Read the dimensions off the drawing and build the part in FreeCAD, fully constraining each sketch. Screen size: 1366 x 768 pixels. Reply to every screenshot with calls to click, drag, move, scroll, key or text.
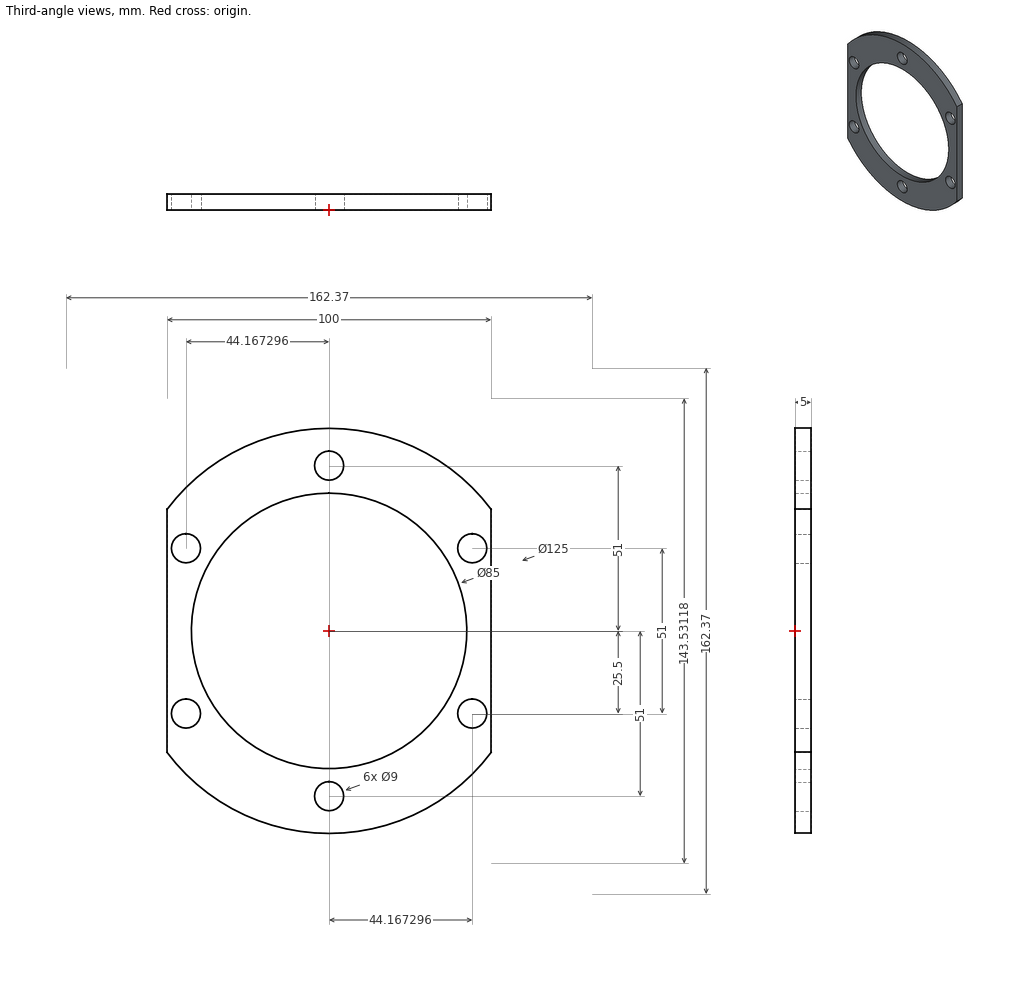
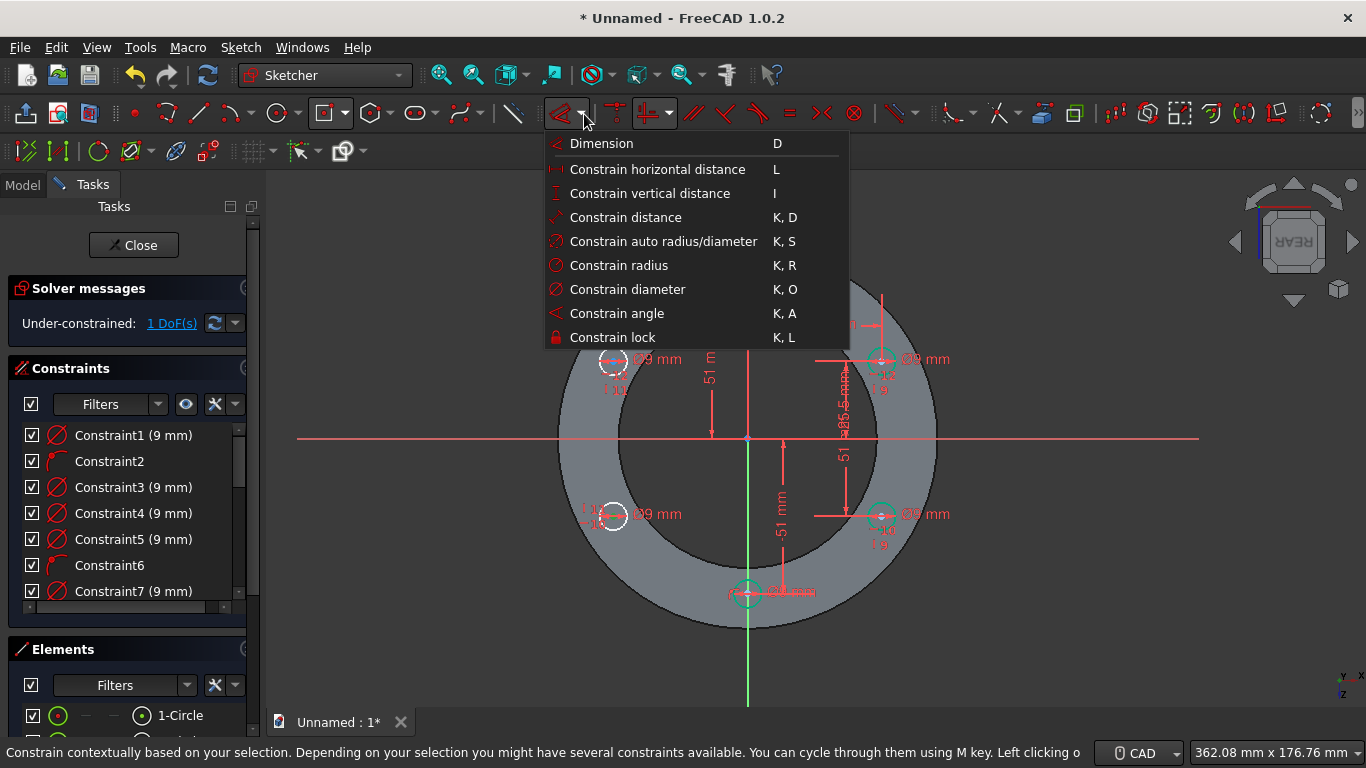
click(697, 169)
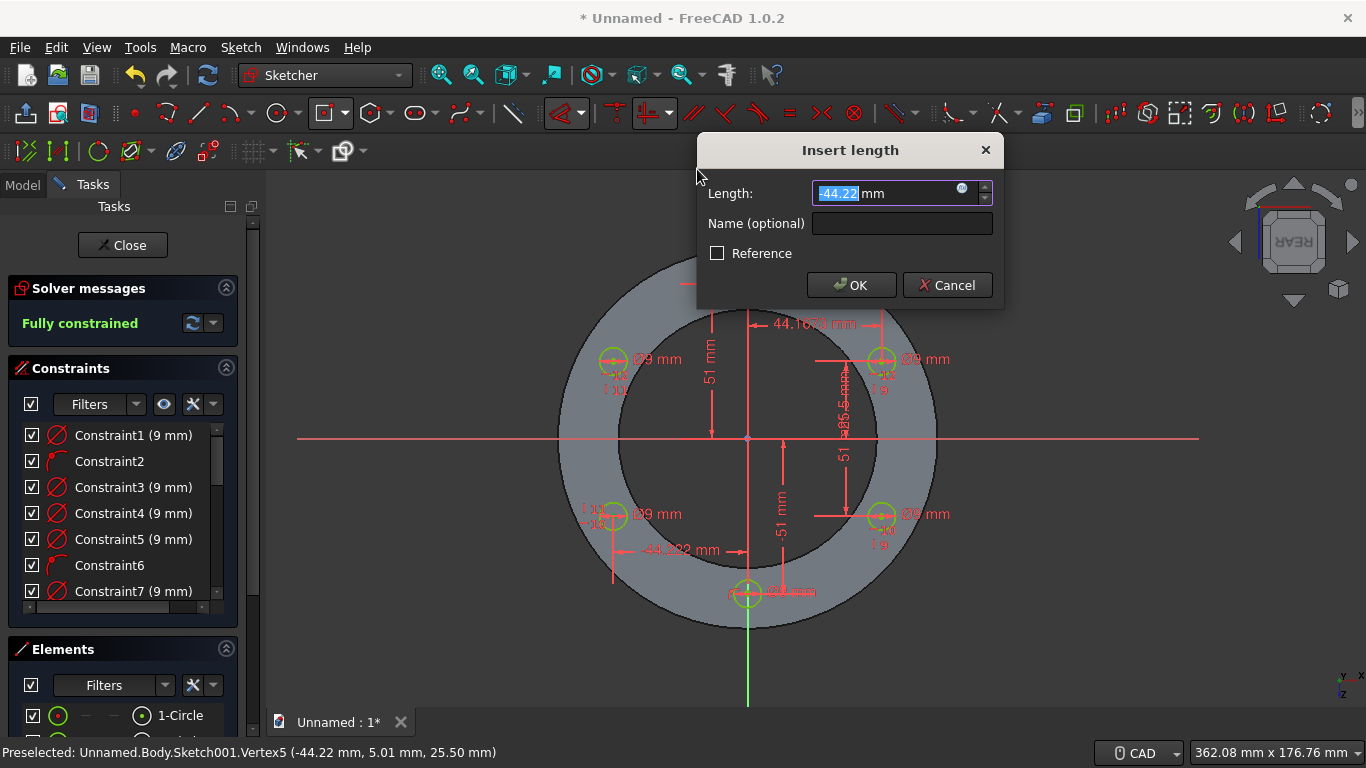
text(-44.167296)
key(Return)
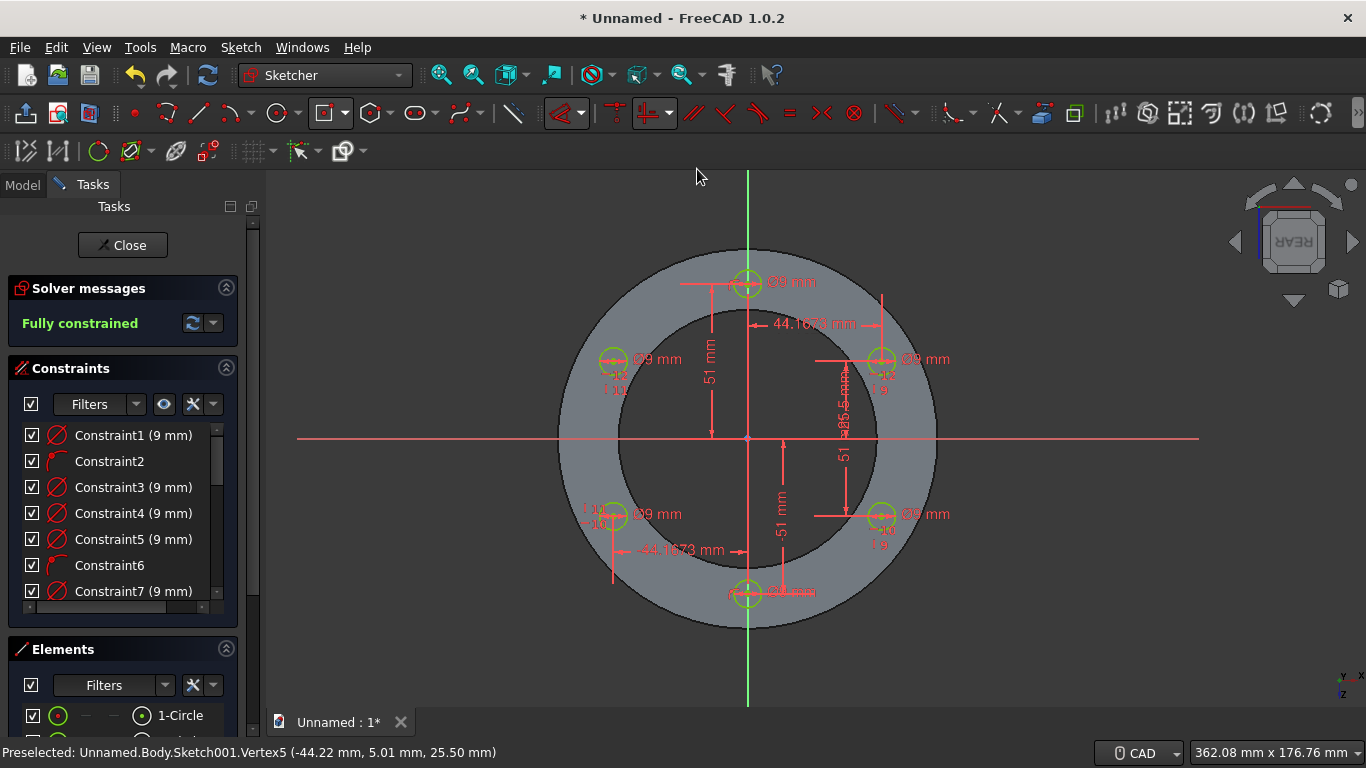
click(123, 245)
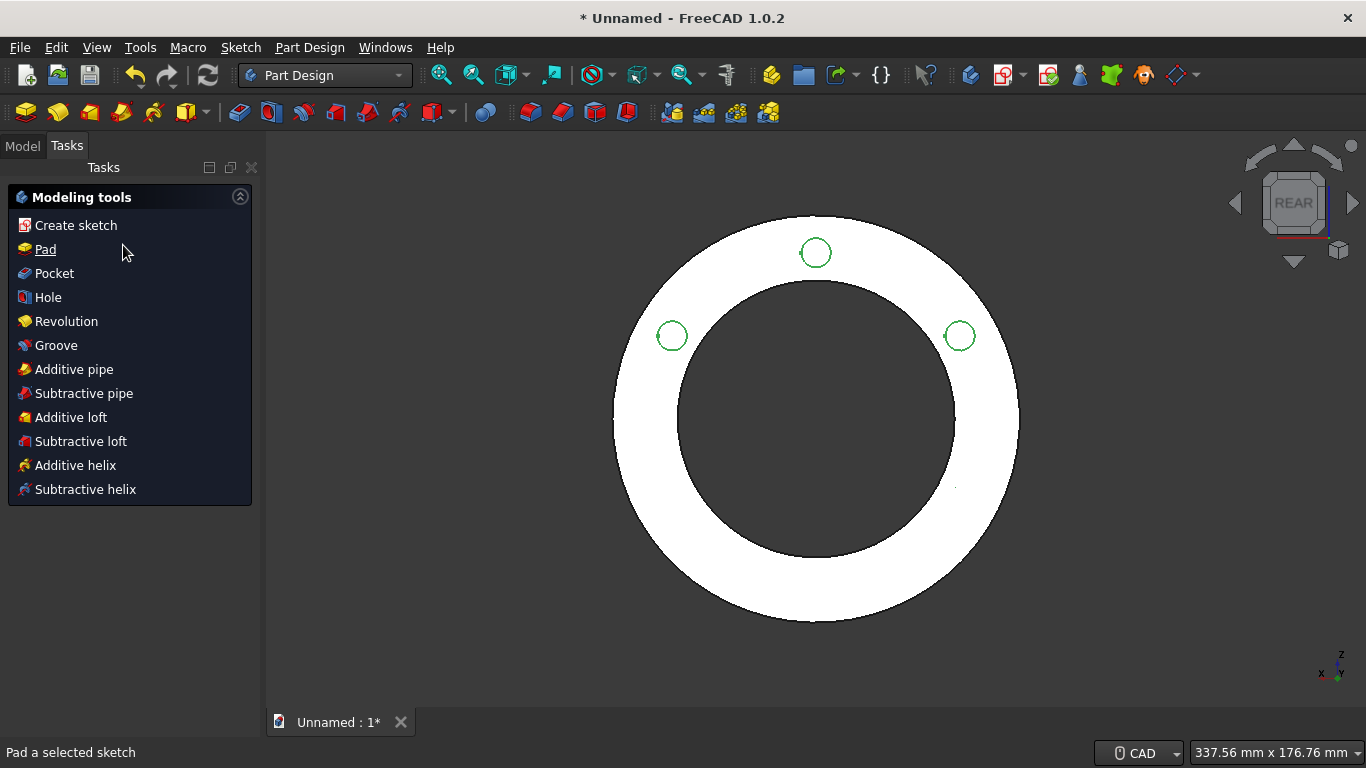
click(240, 112)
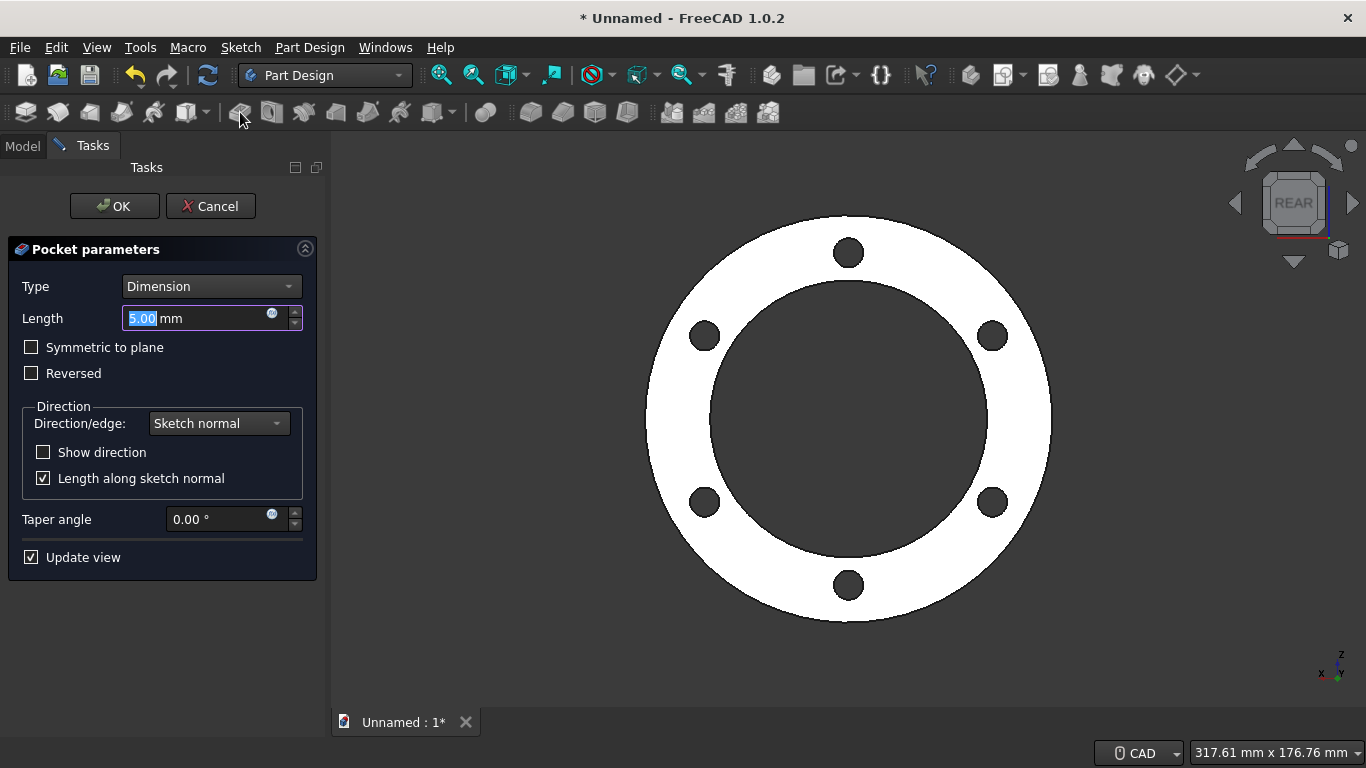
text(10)
key(Tab)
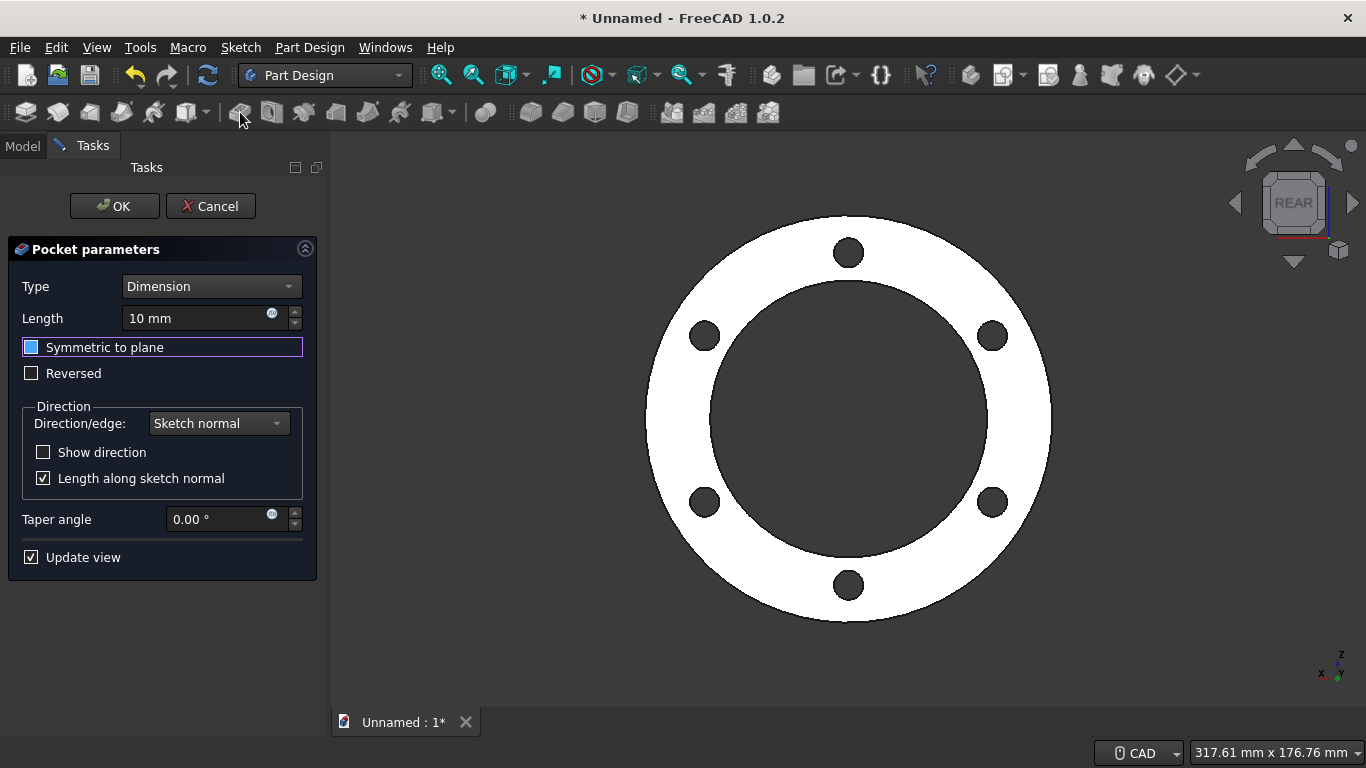
click(115, 206)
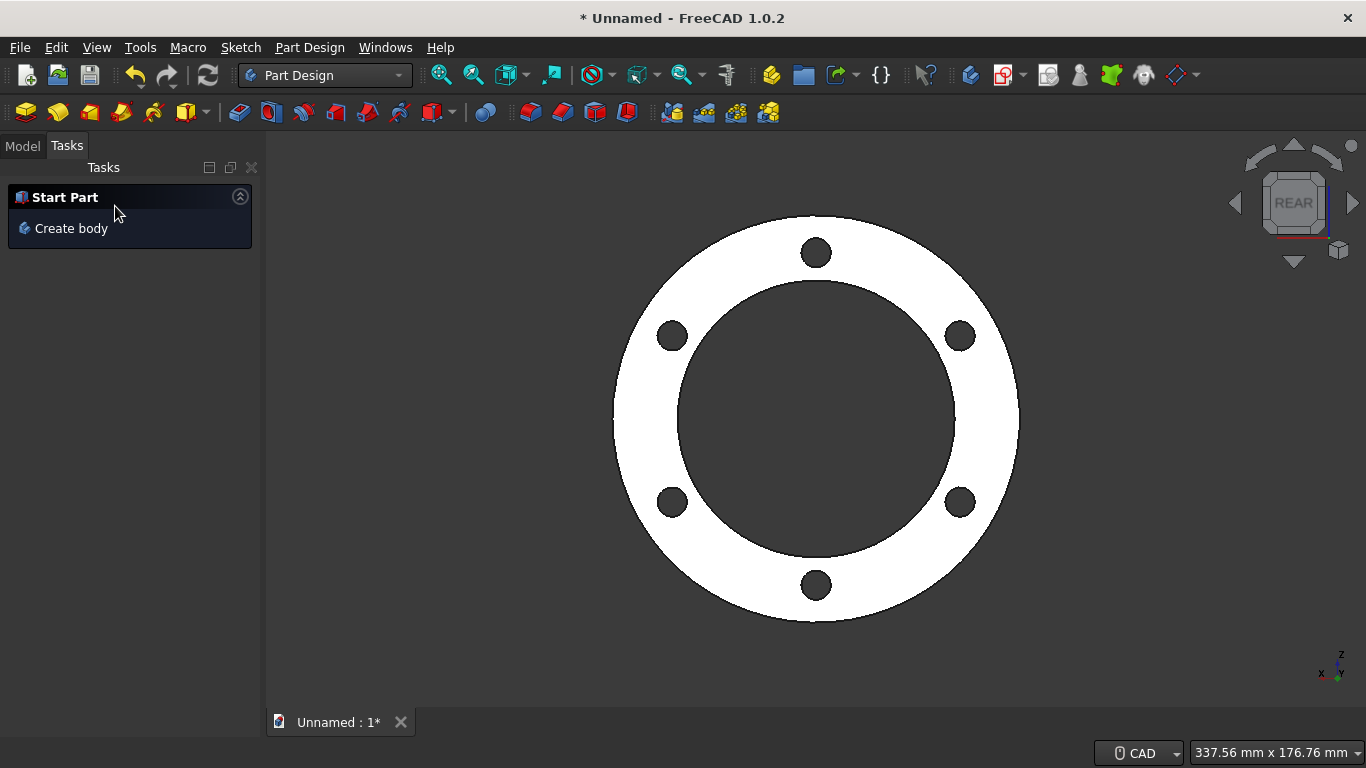
click(642, 418)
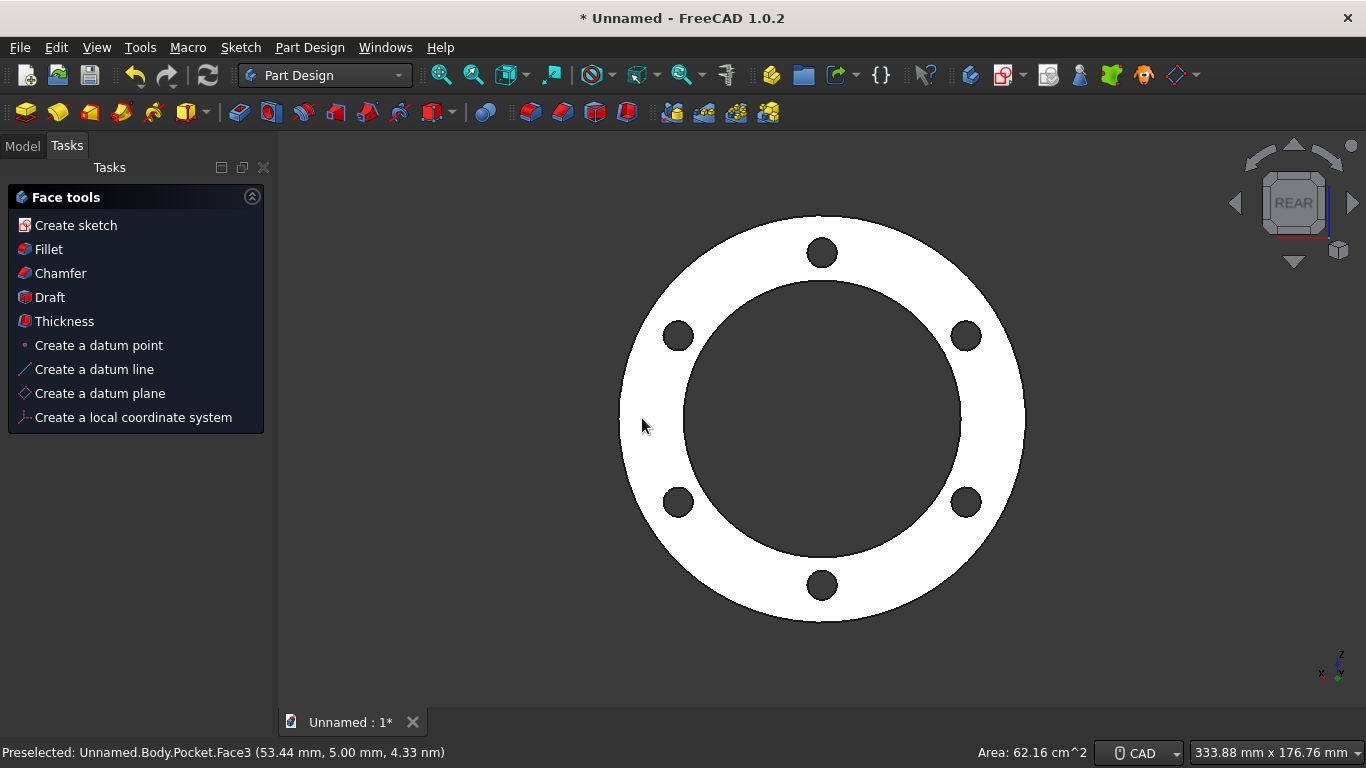
click(1004, 76)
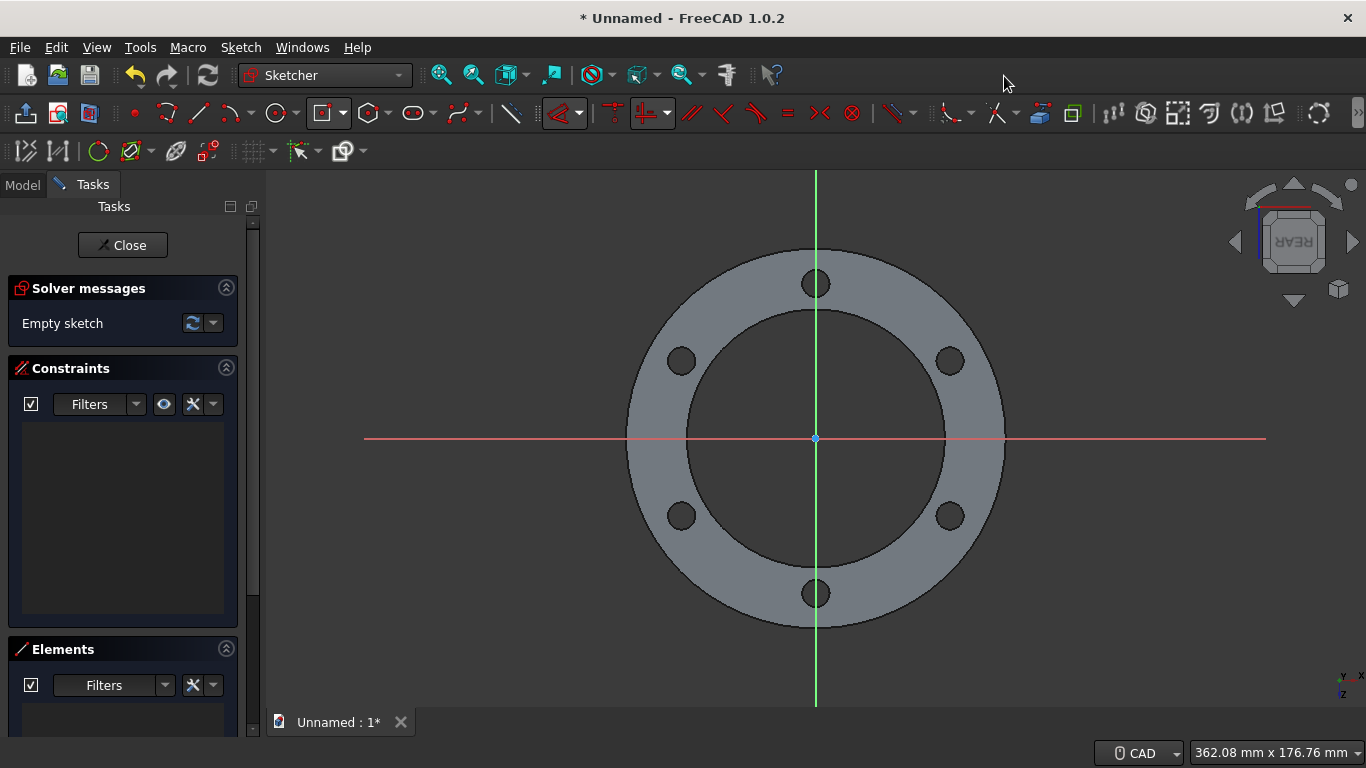
scroll(608, 439, down, 2)